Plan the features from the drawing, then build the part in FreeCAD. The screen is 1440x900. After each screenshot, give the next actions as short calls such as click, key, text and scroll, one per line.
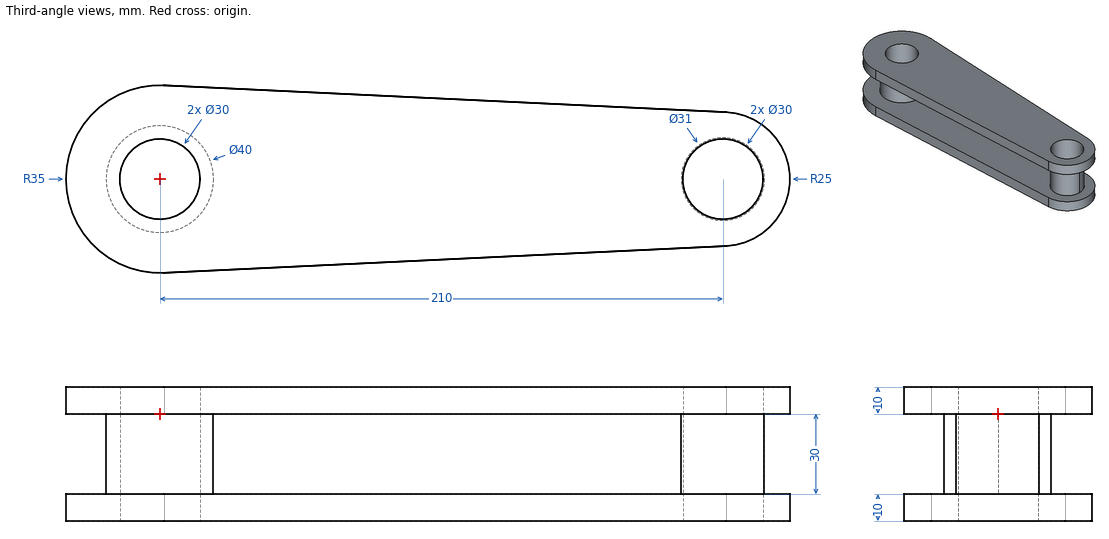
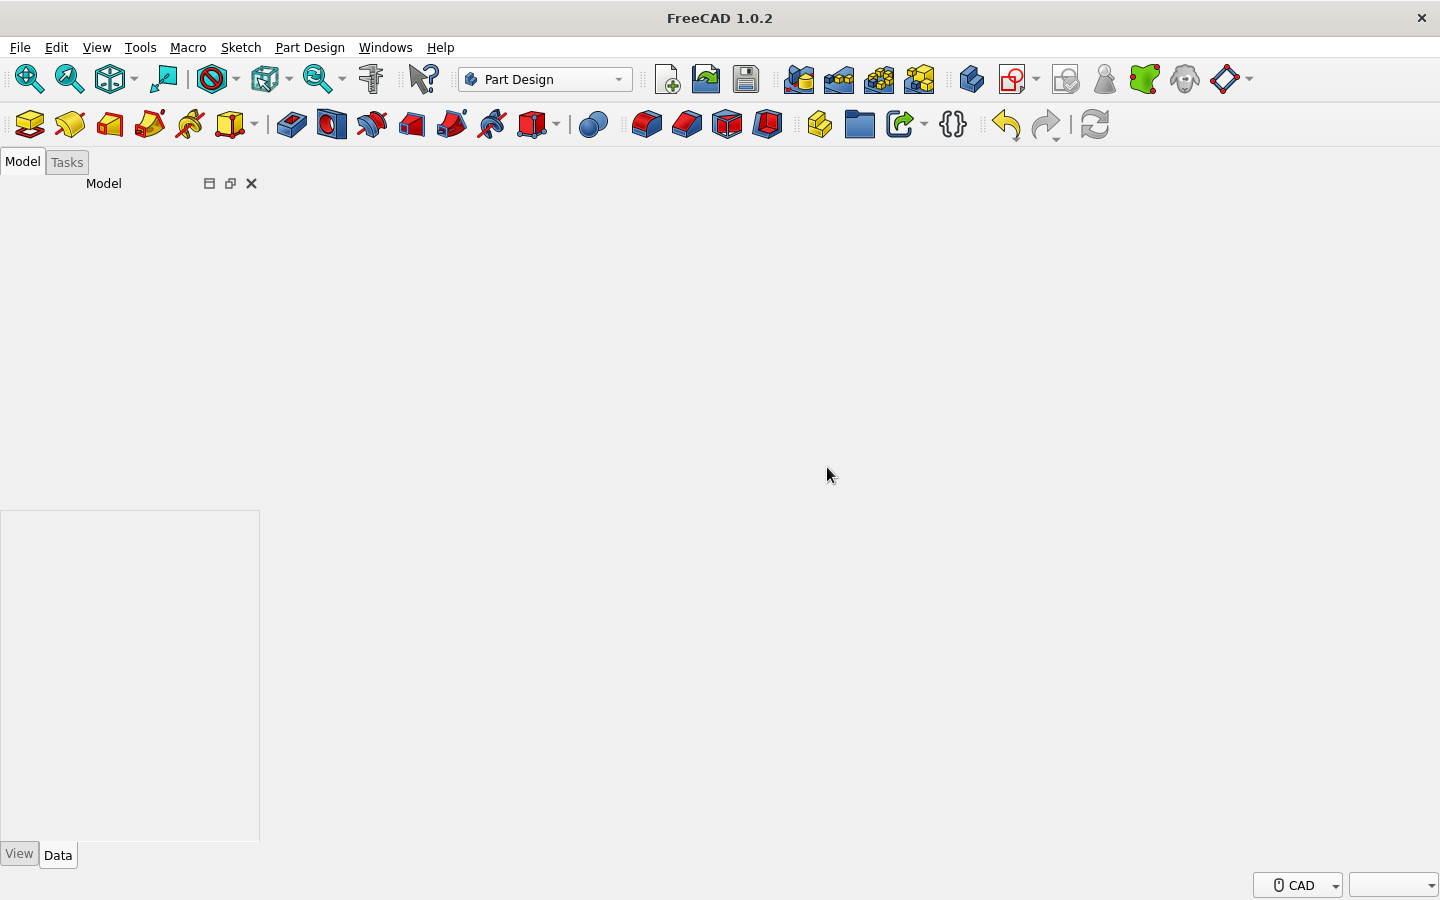
click(666, 80)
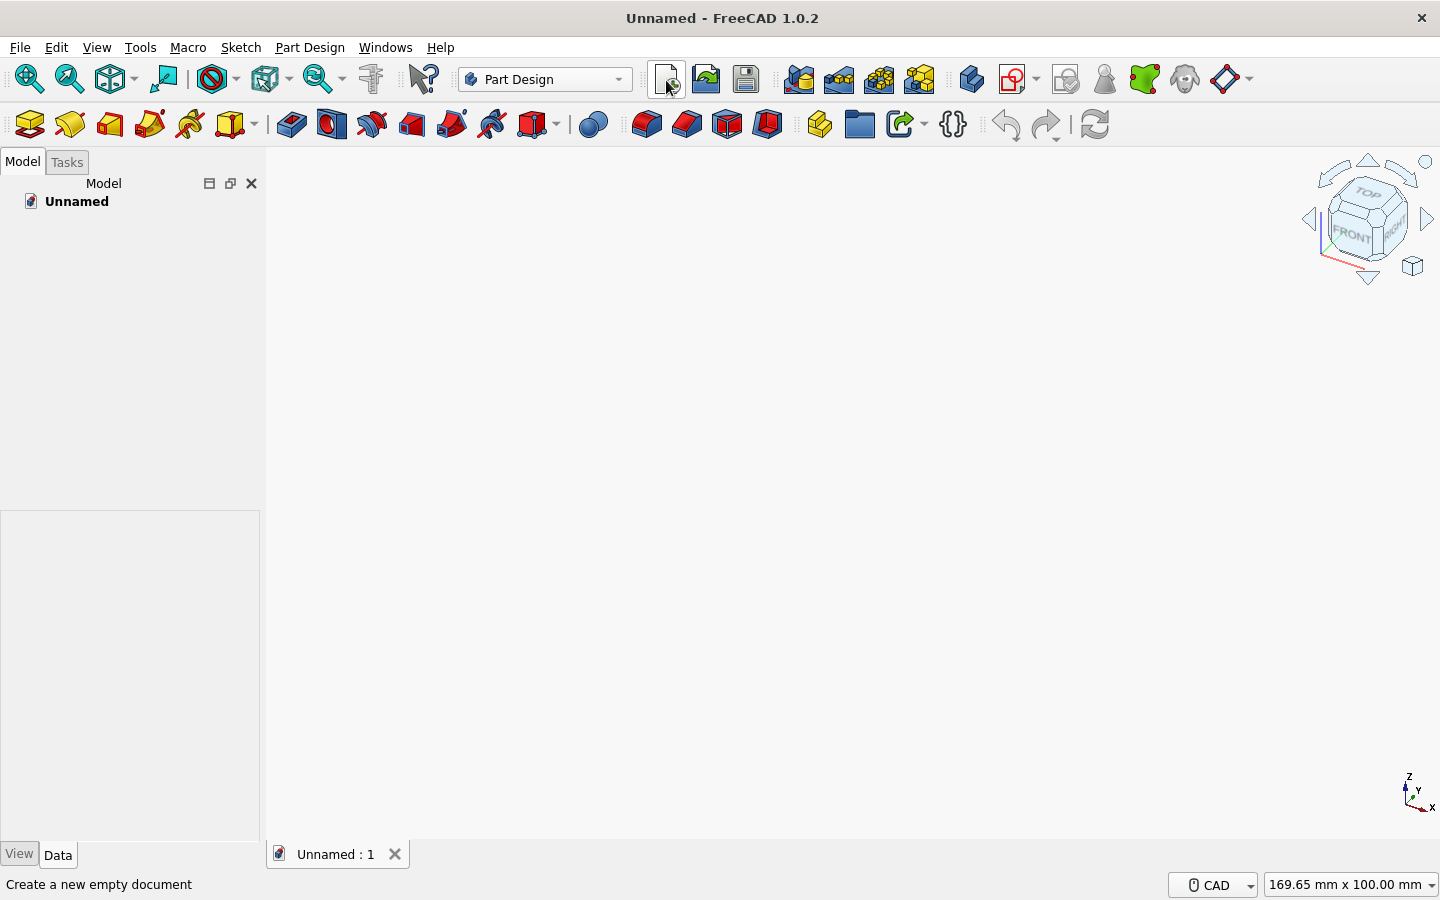
click(1012, 80)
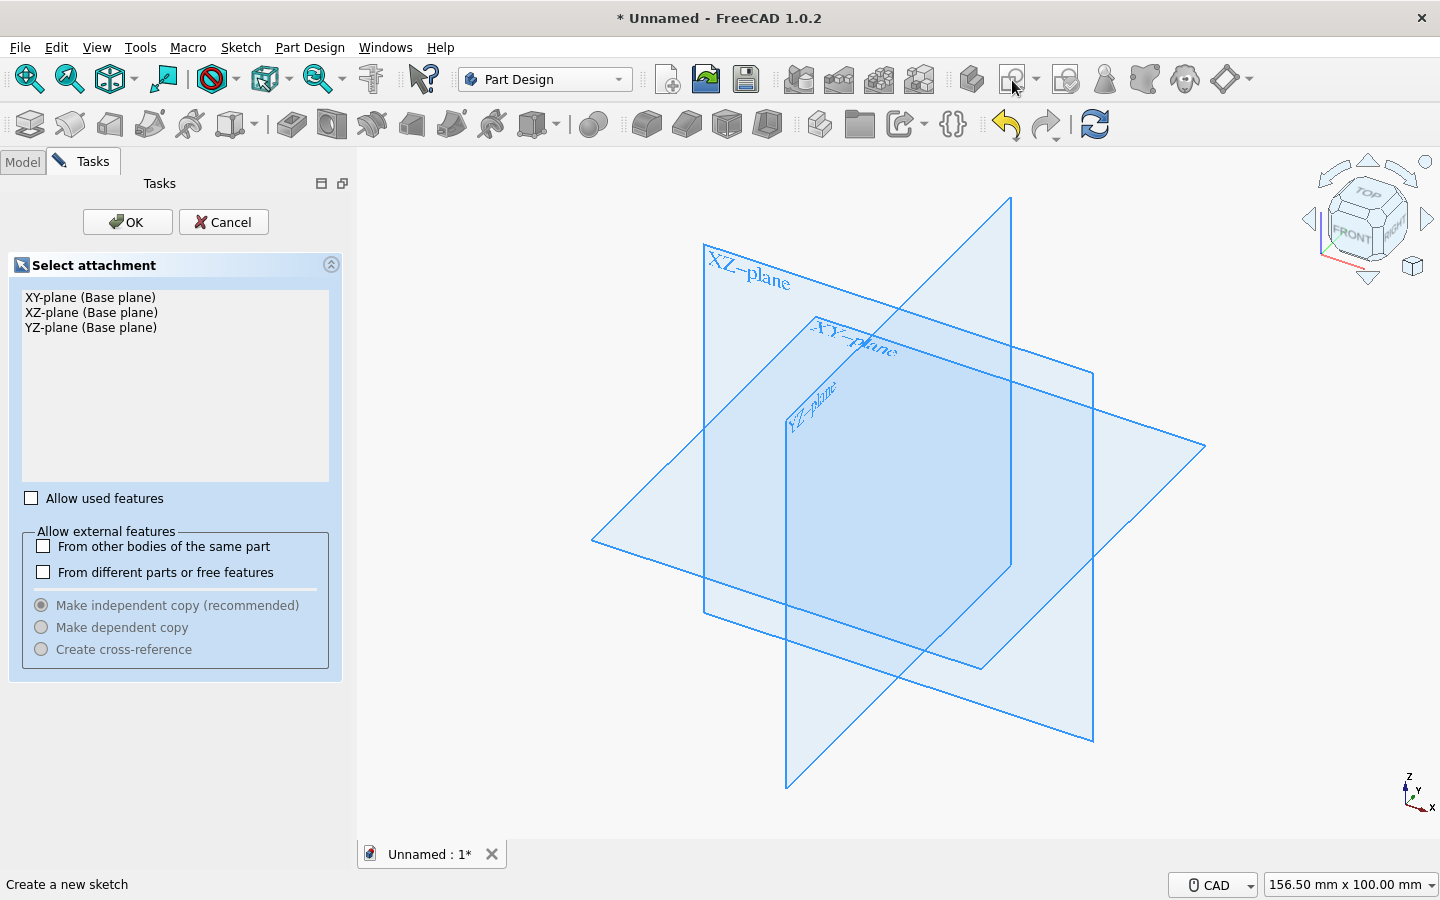
click(82, 298)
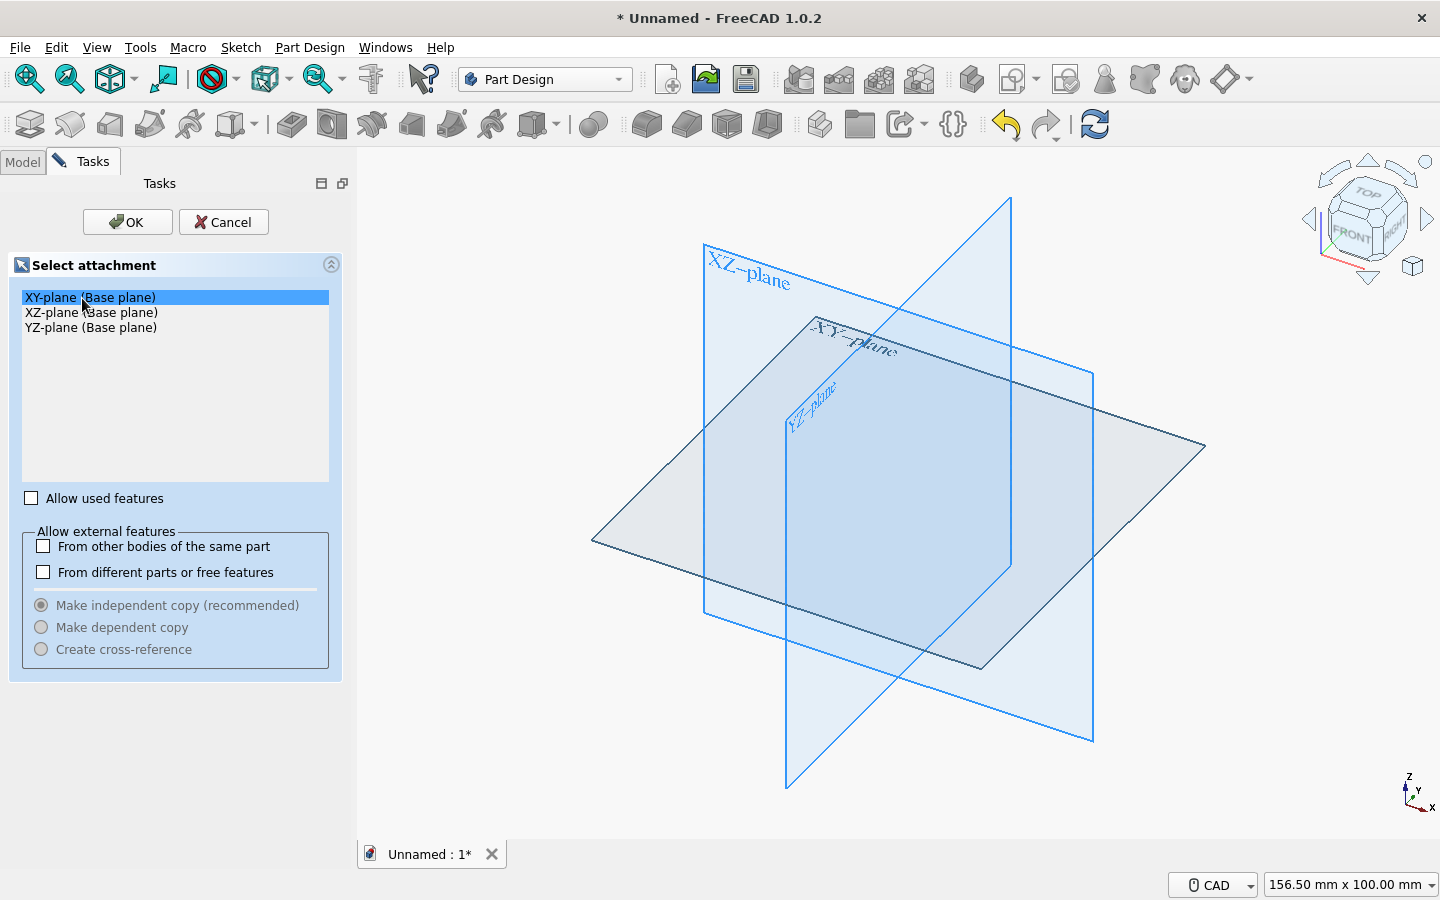
click(128, 222)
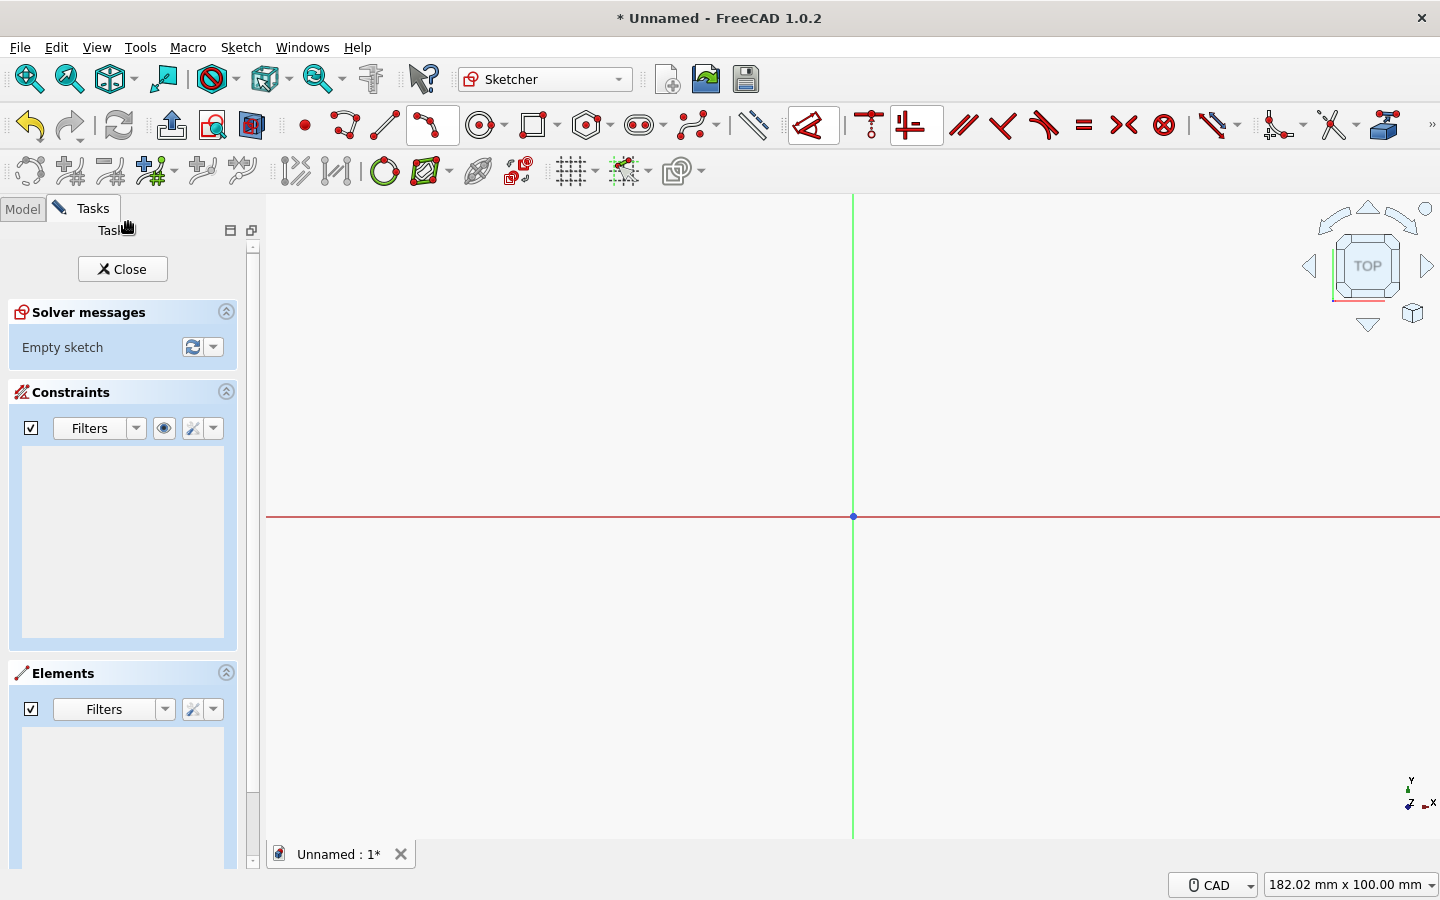
scroll(369, 516, down, 5)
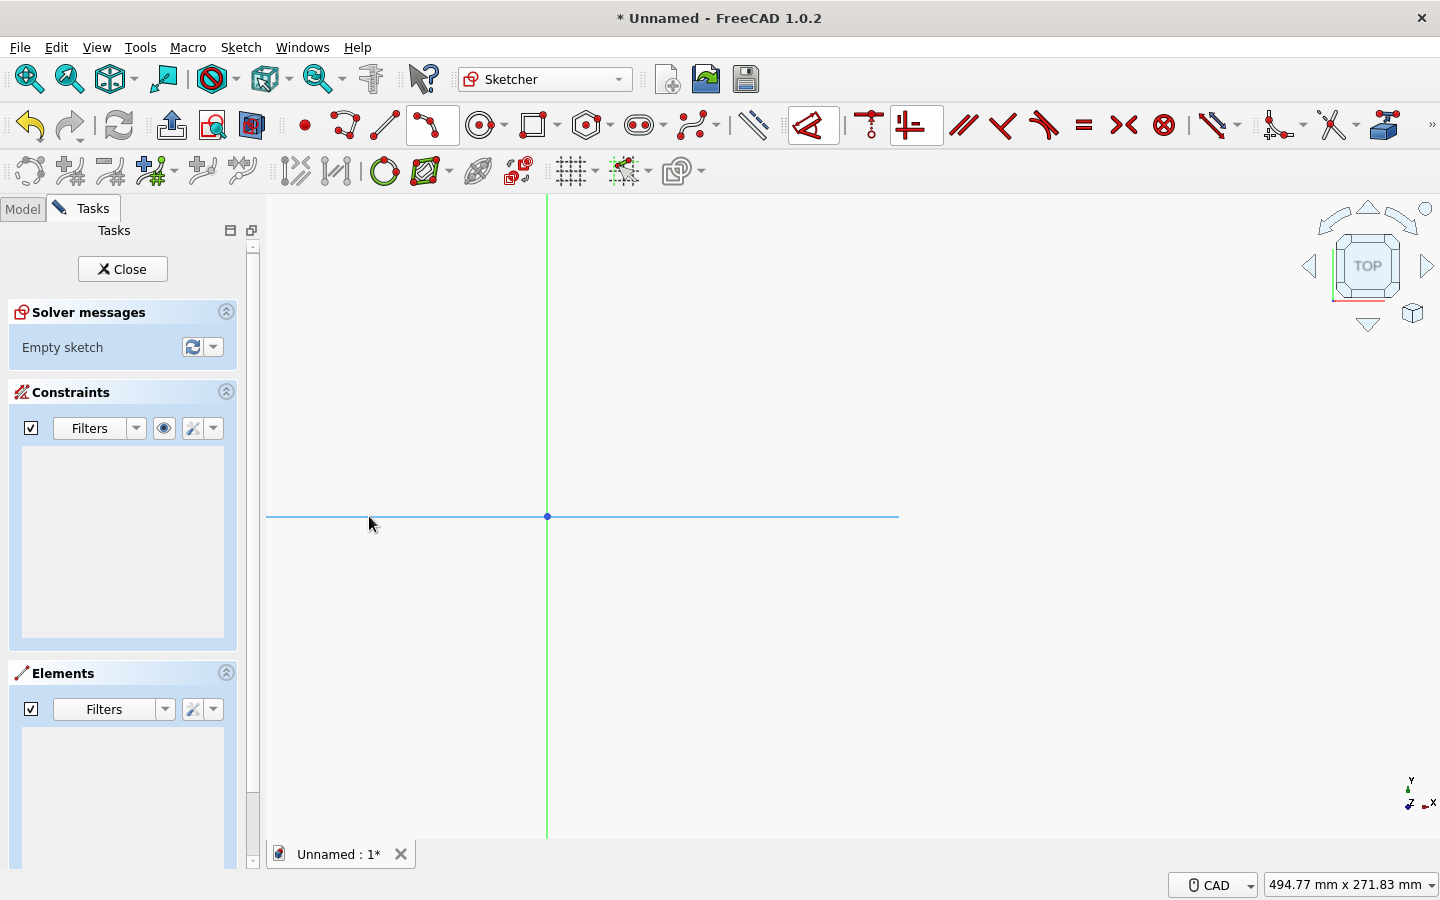
click(386, 126)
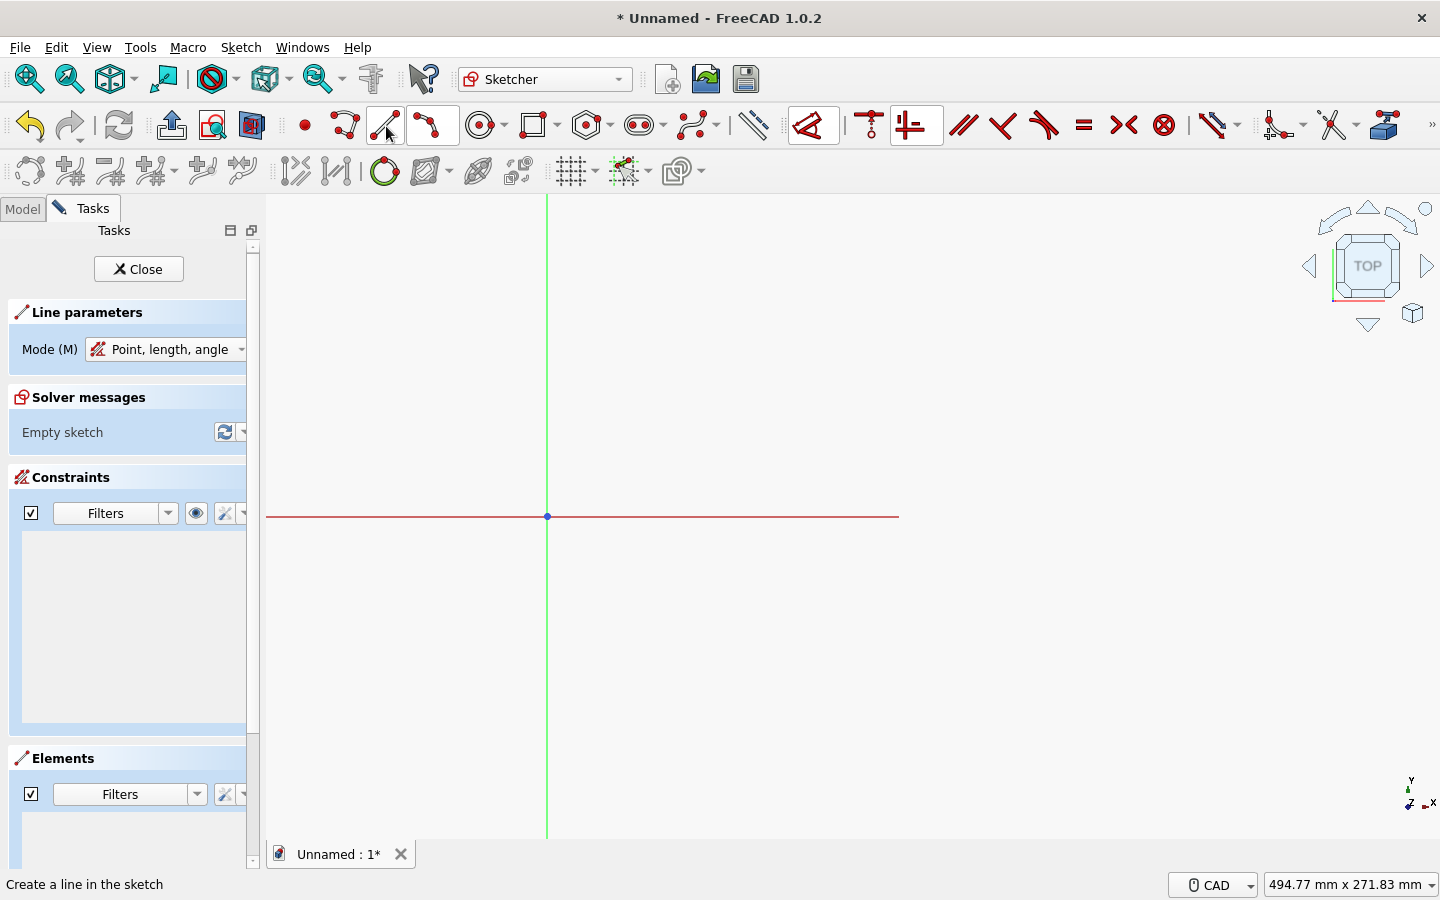
click(1048, 457)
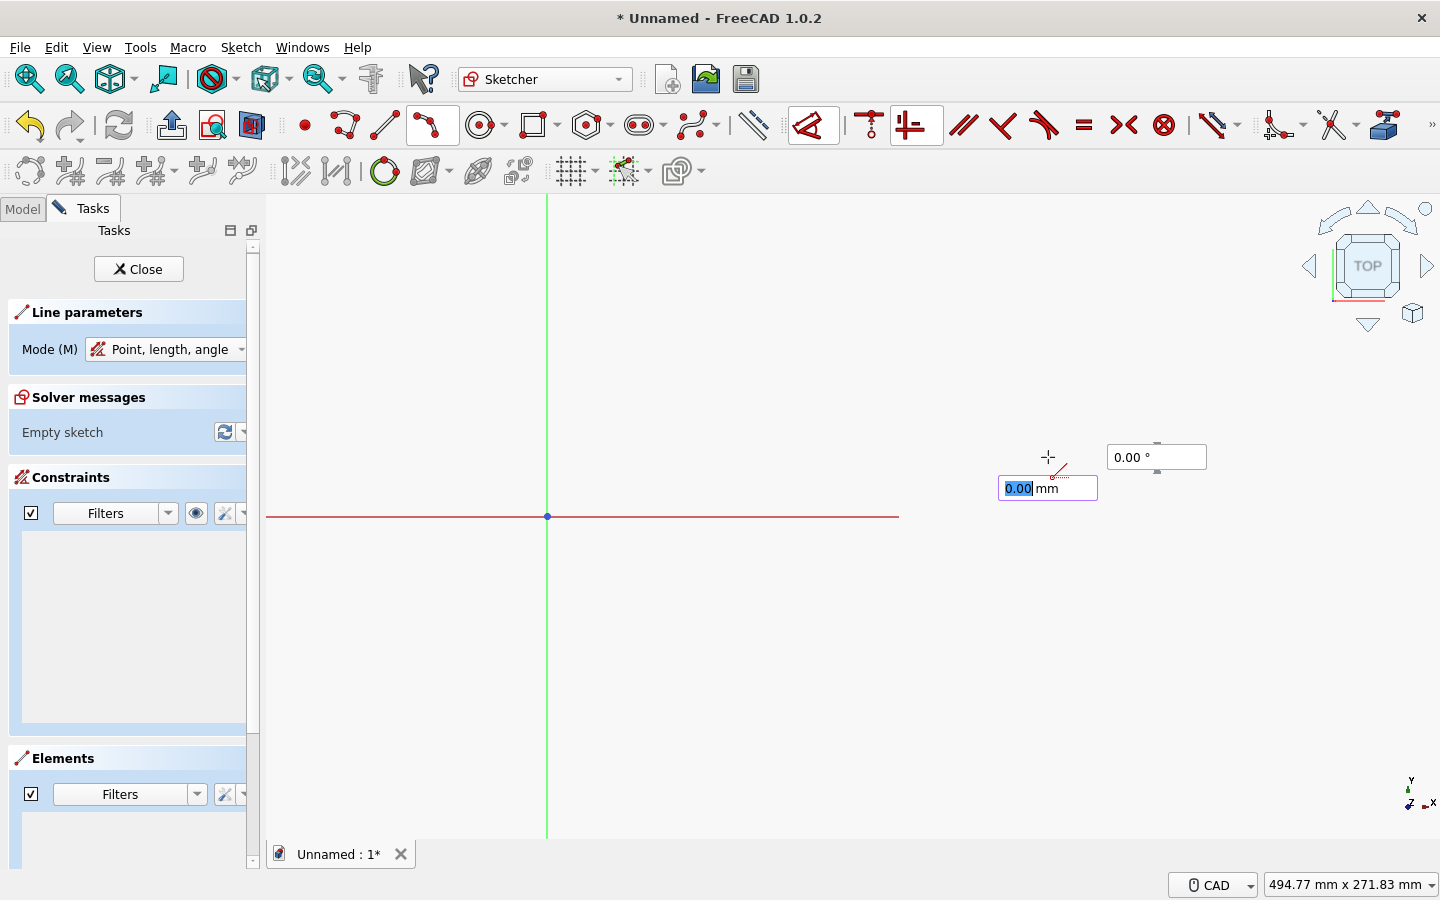
scroll(551, 434, up, 7)